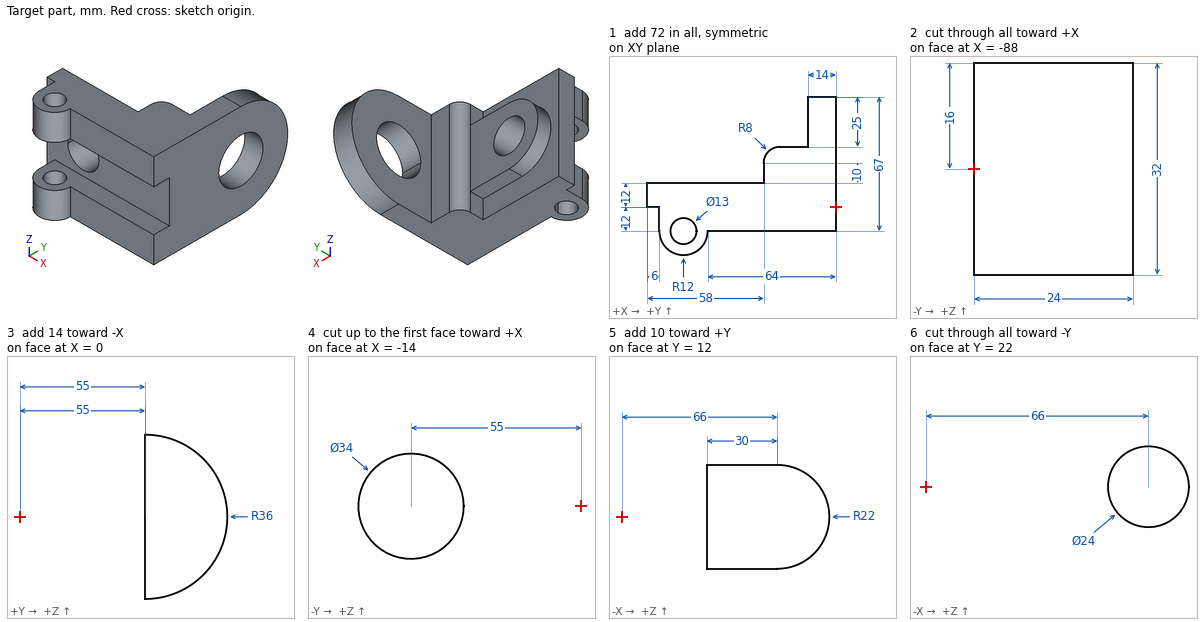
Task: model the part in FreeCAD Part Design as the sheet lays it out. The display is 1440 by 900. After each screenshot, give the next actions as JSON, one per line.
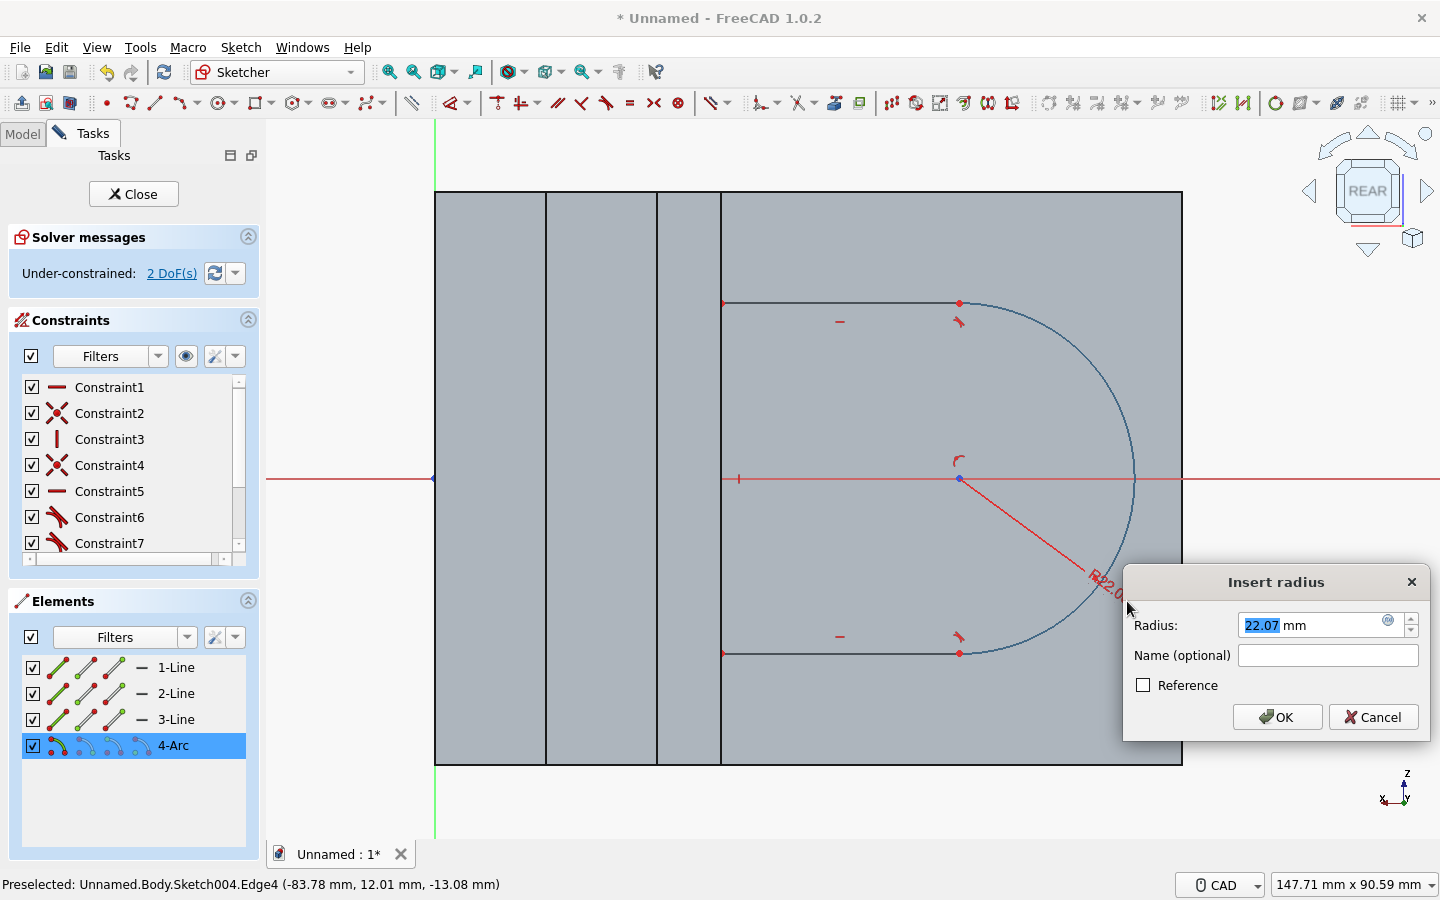
{"action": "type", "text": "22"}
{"action": "key", "text": "Return"}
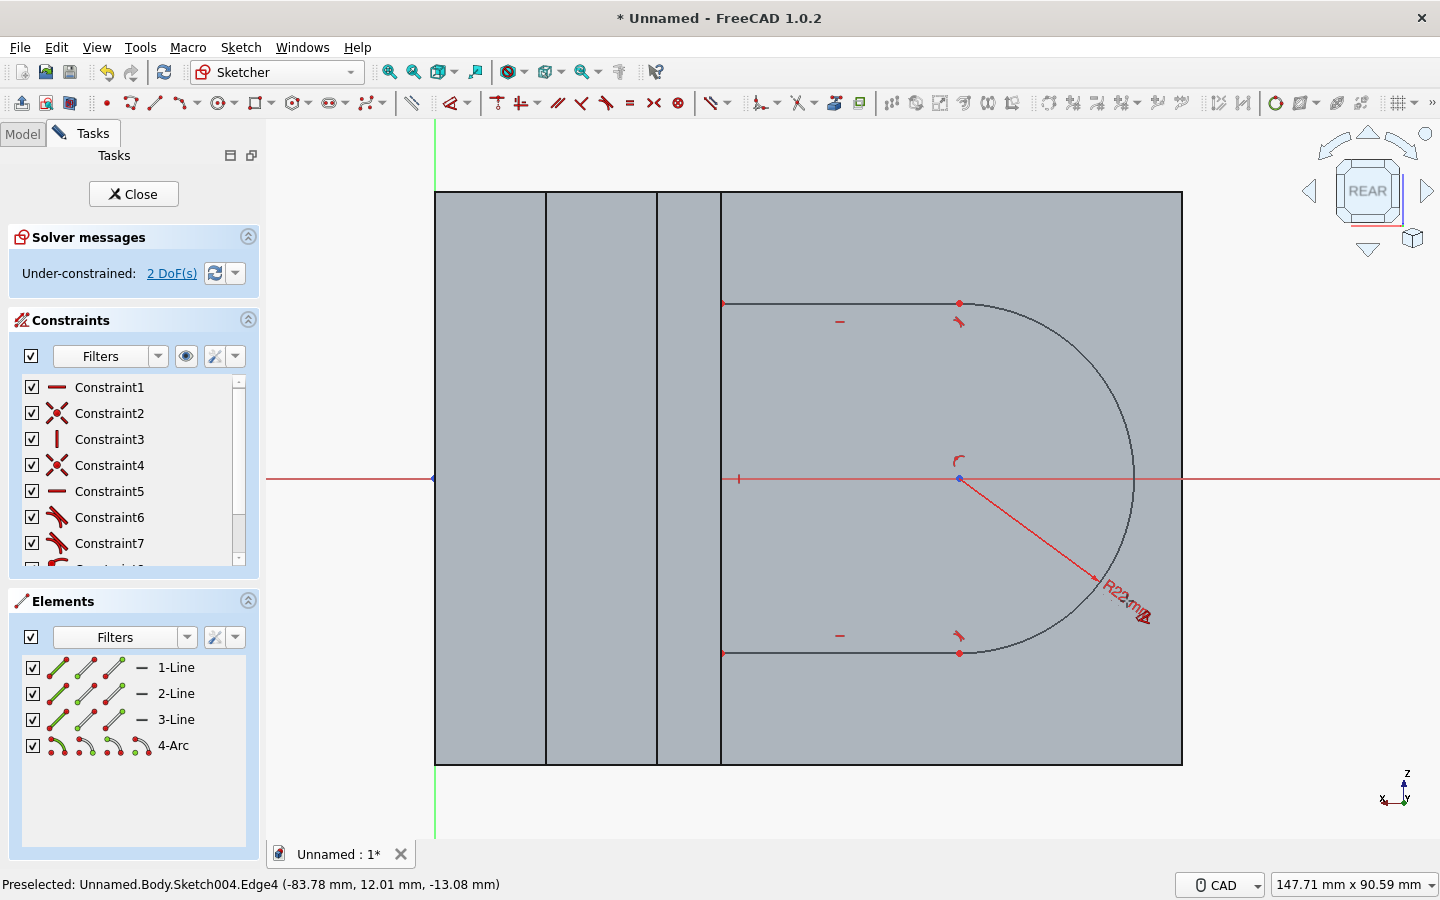
{"action": "left_click", "coordinate": [888, 304]}
{"action": "left_click", "coordinate": [840, 270]}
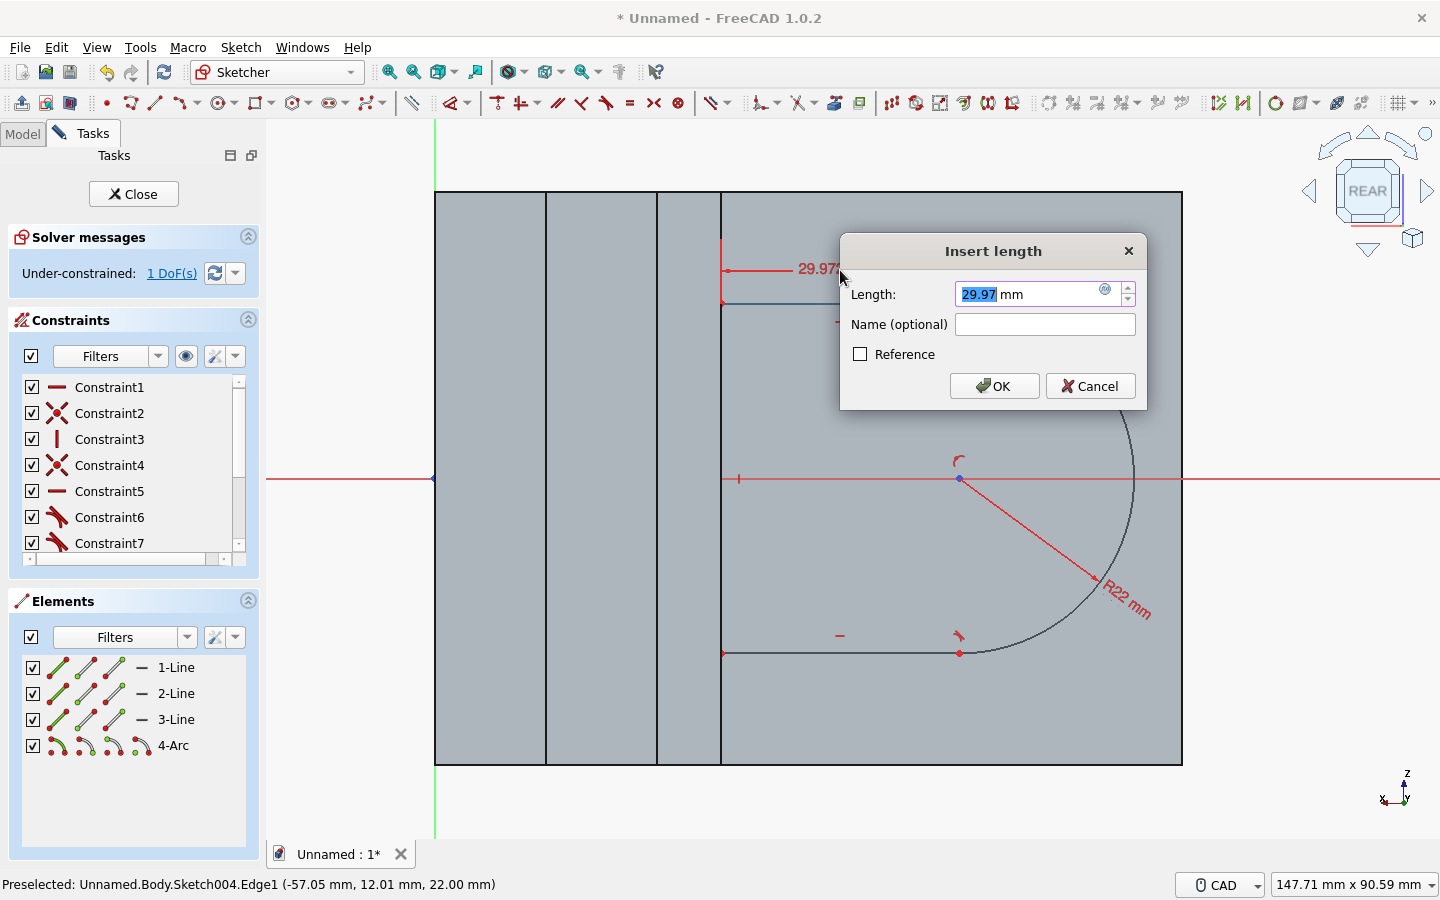
{"action": "type", "text": "30"}
{"action": "key", "text": "Return"}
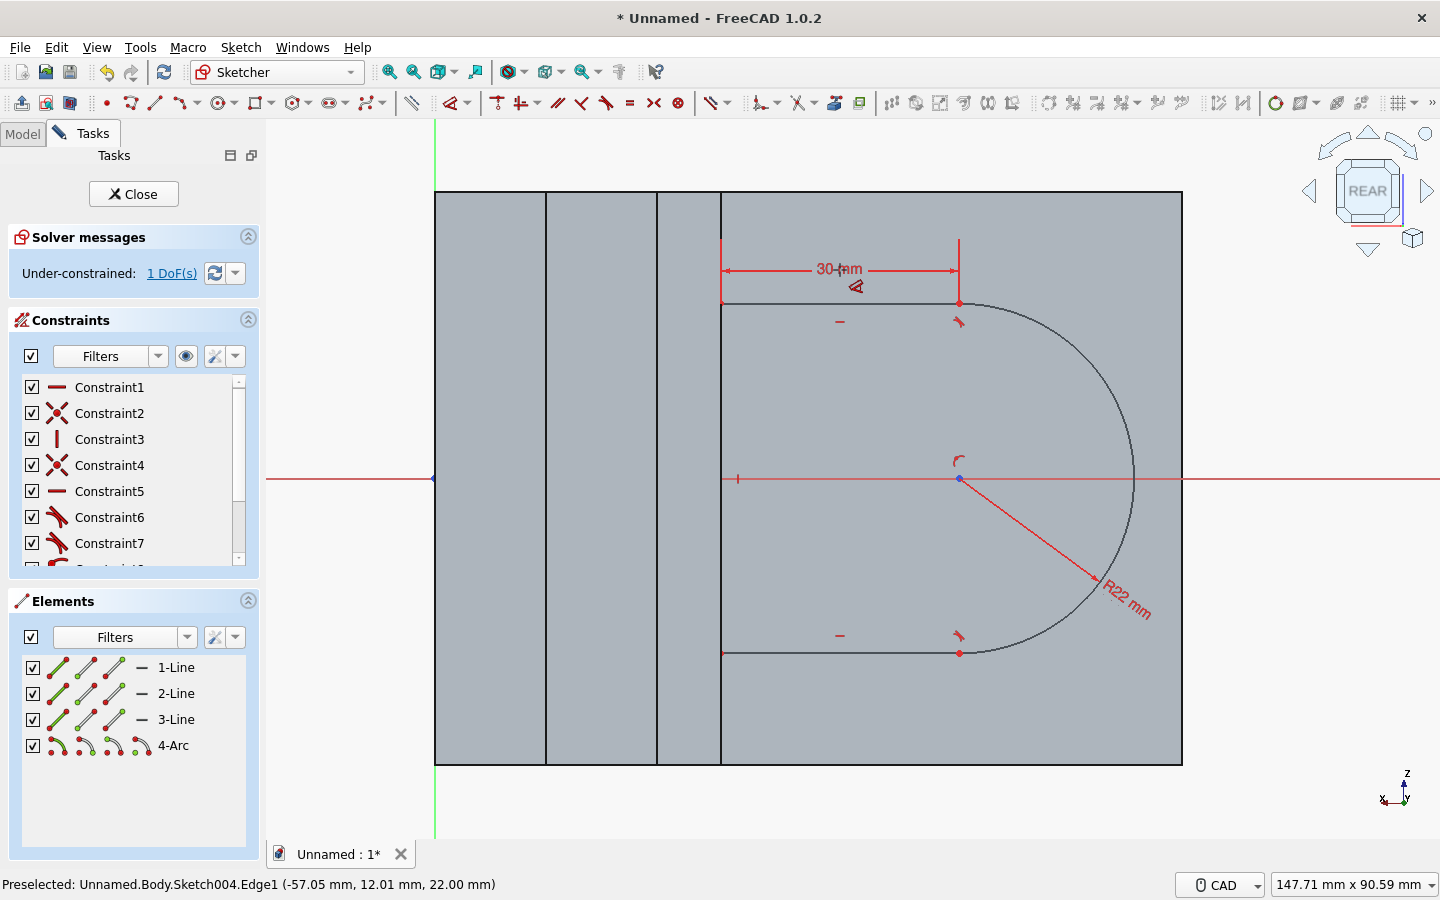
{"action": "left_click", "coordinate": [959, 304]}
{"action": "left_click", "coordinate": [697, 270]}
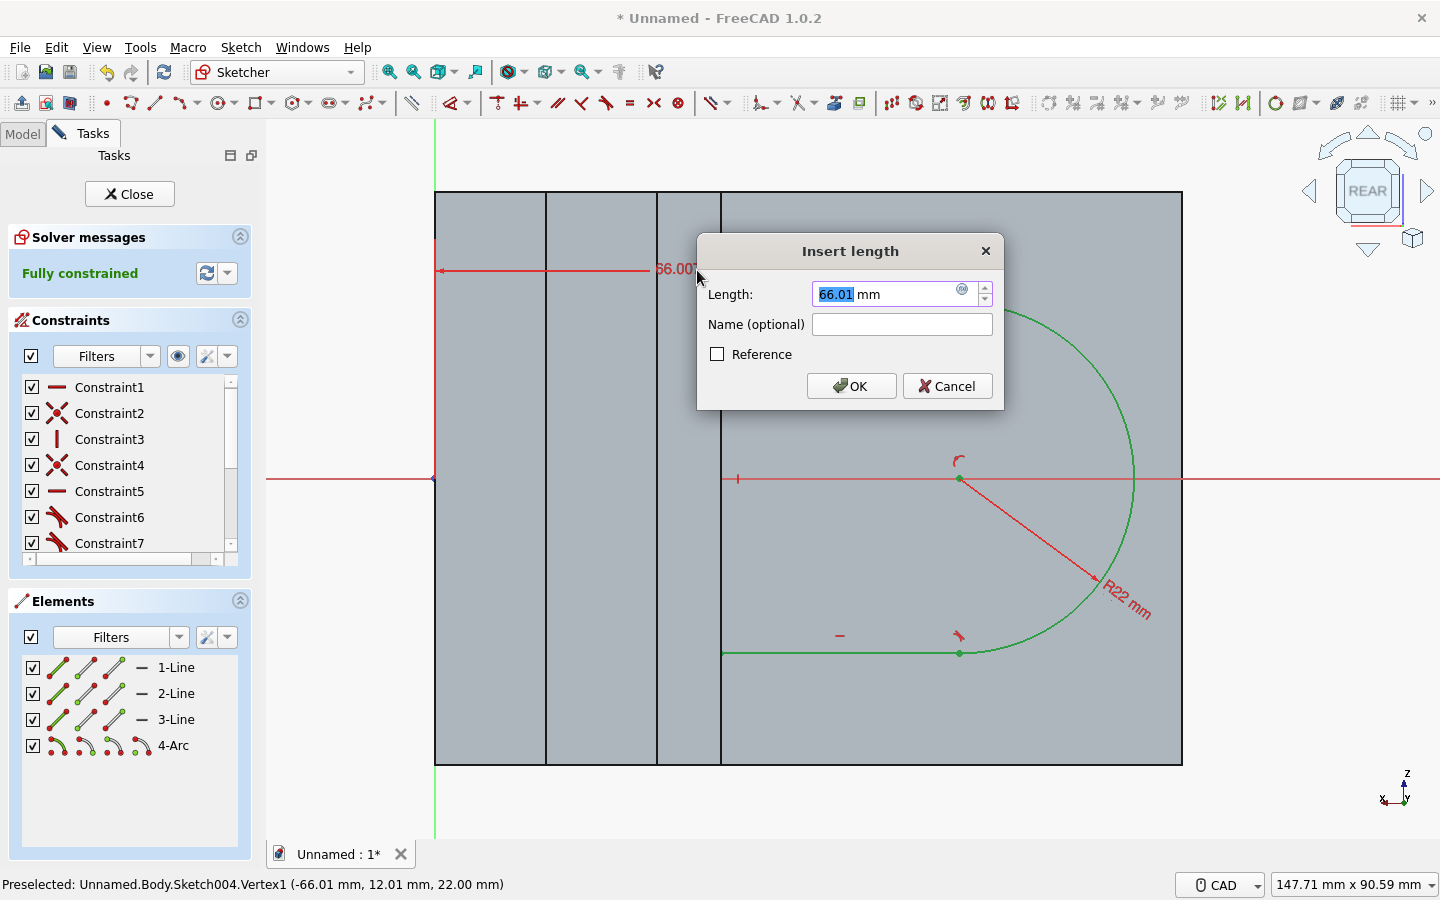
{"action": "type", "text": "66"}
{"action": "key", "text": "Return"}
{"action": "key", "text": "Escape"}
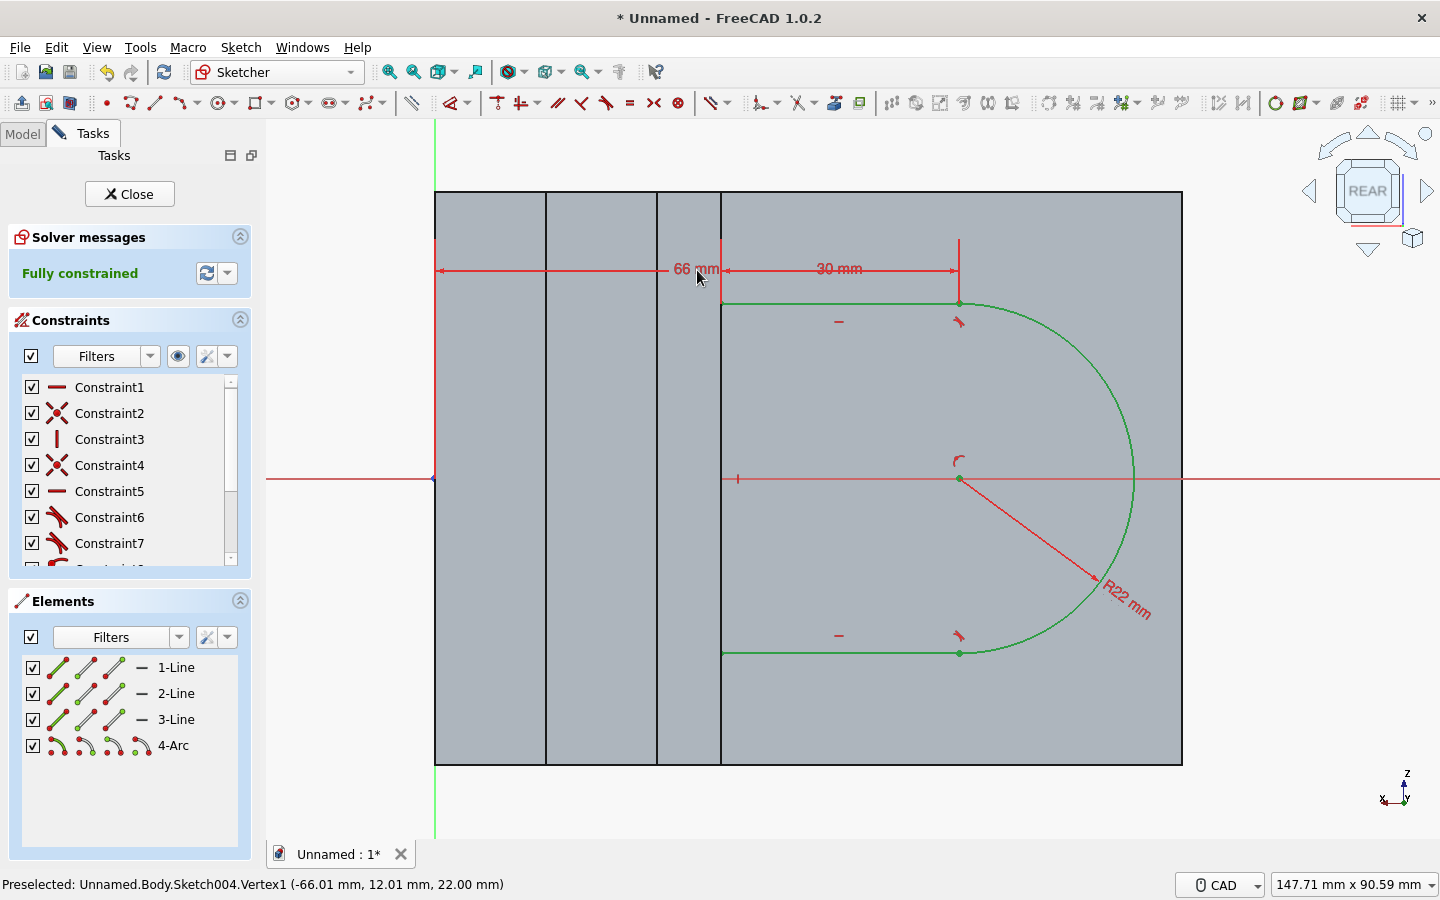
{"action": "left_click", "coordinate": [130, 194]}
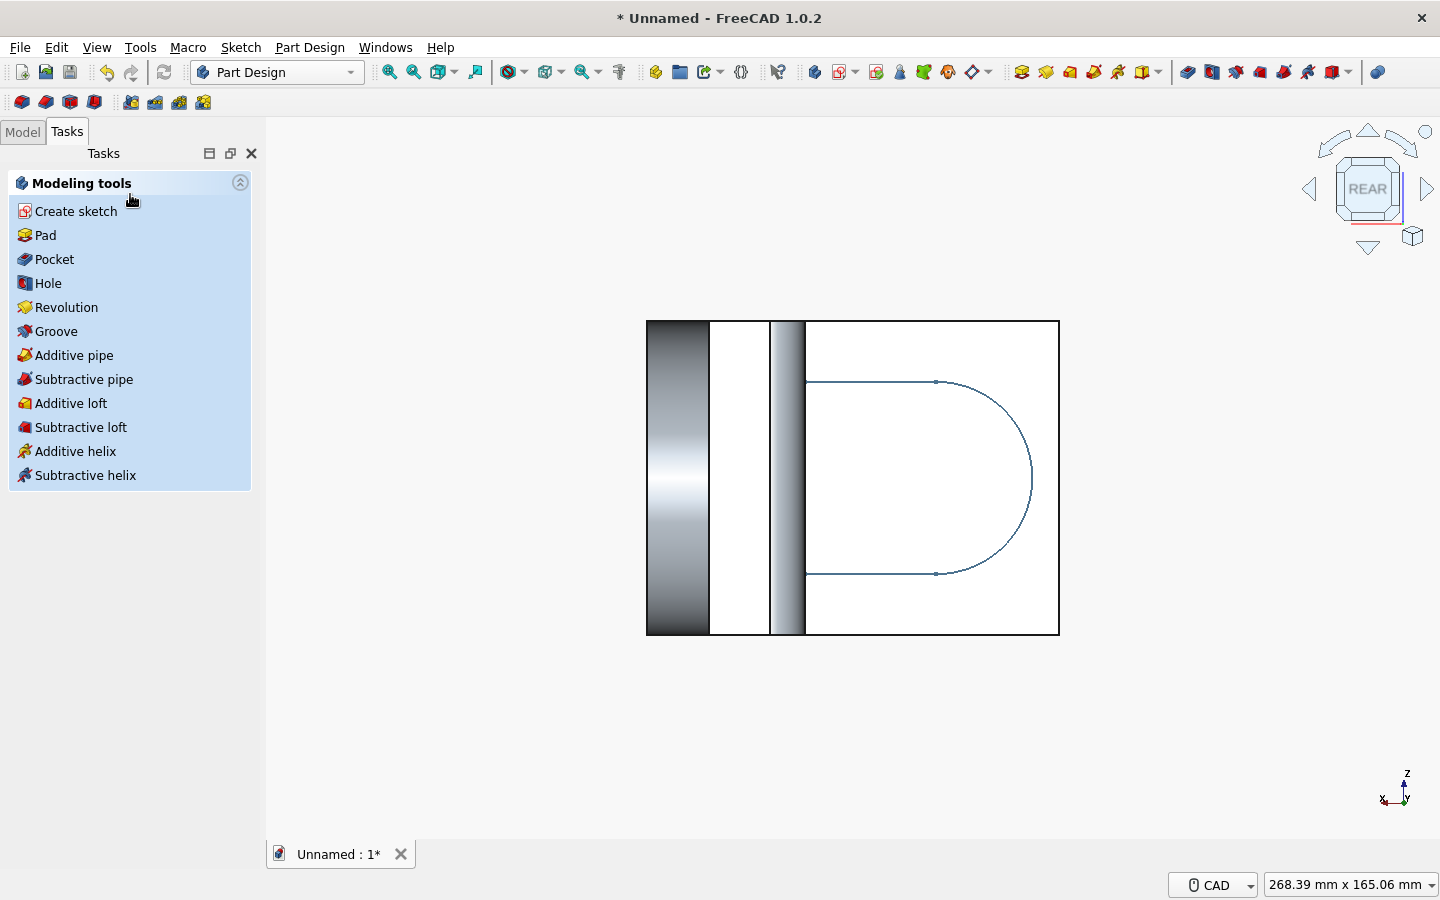
{"action": "left_click", "coordinate": [1022, 72]}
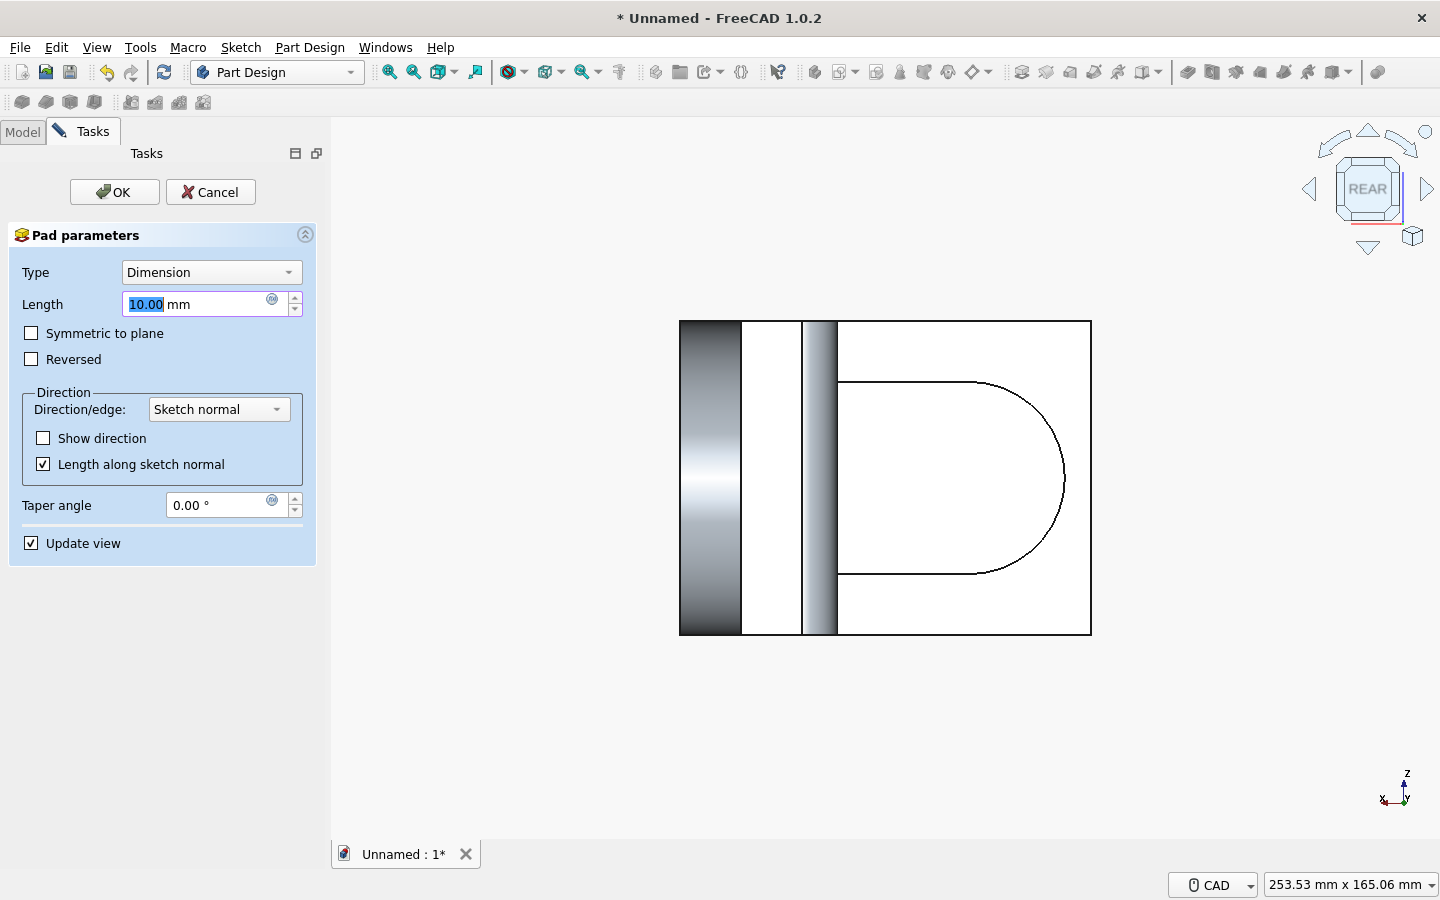
{"action": "type", "text": "10"}
{"action": "key", "text": "Tab"}